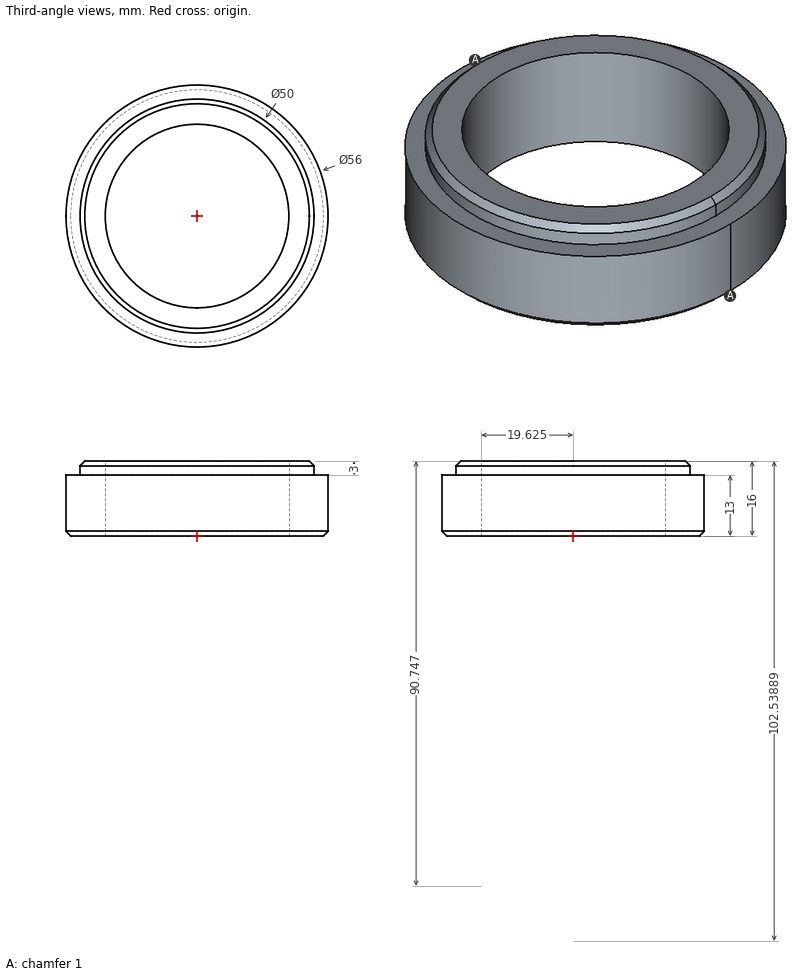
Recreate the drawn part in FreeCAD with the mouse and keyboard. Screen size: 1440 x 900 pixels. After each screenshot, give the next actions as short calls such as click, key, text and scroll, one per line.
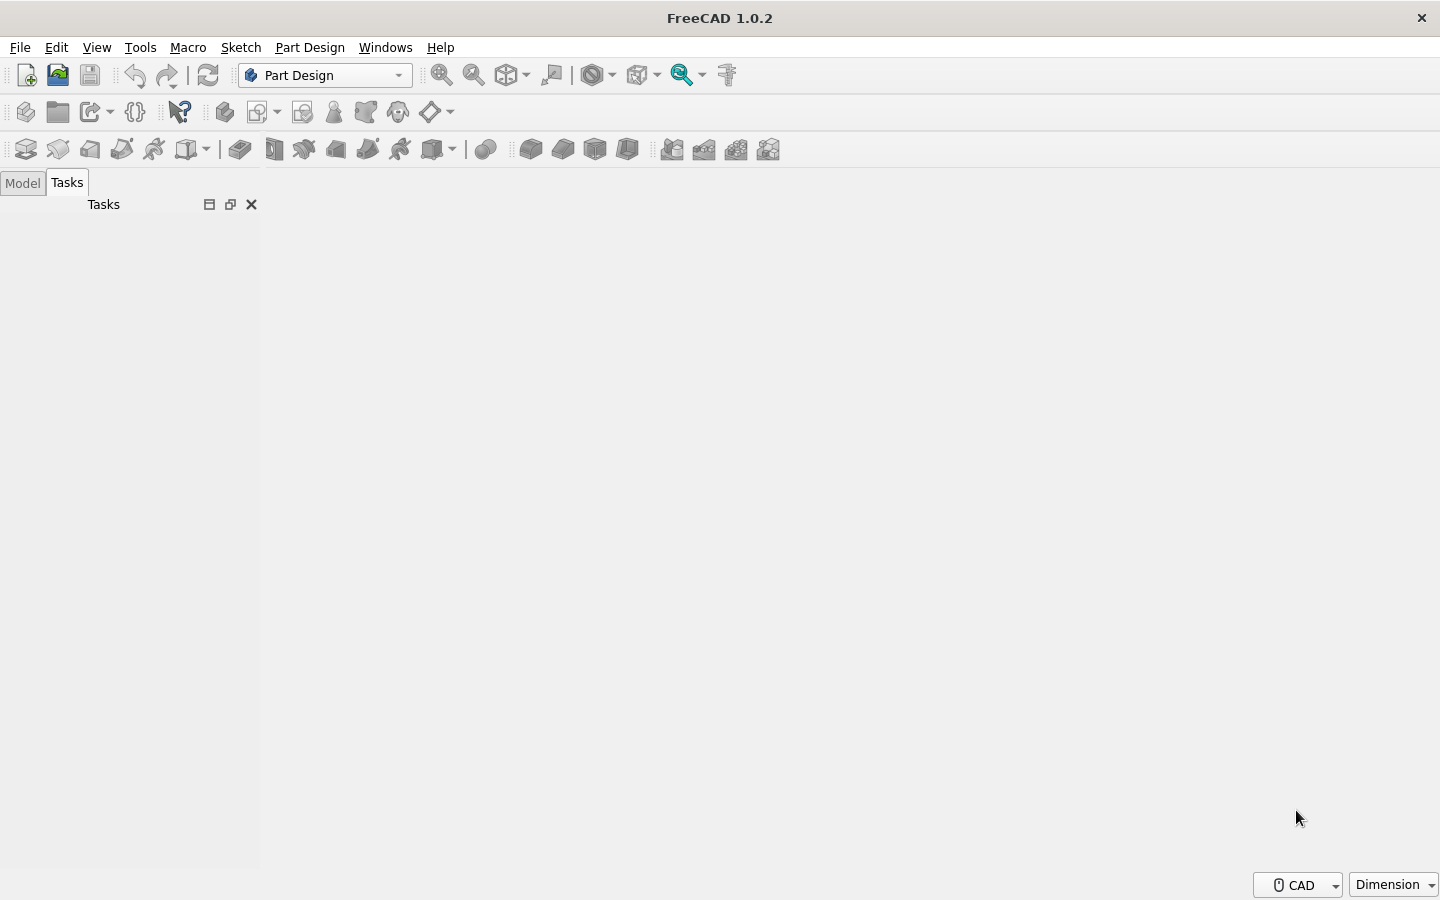
click(290, 76)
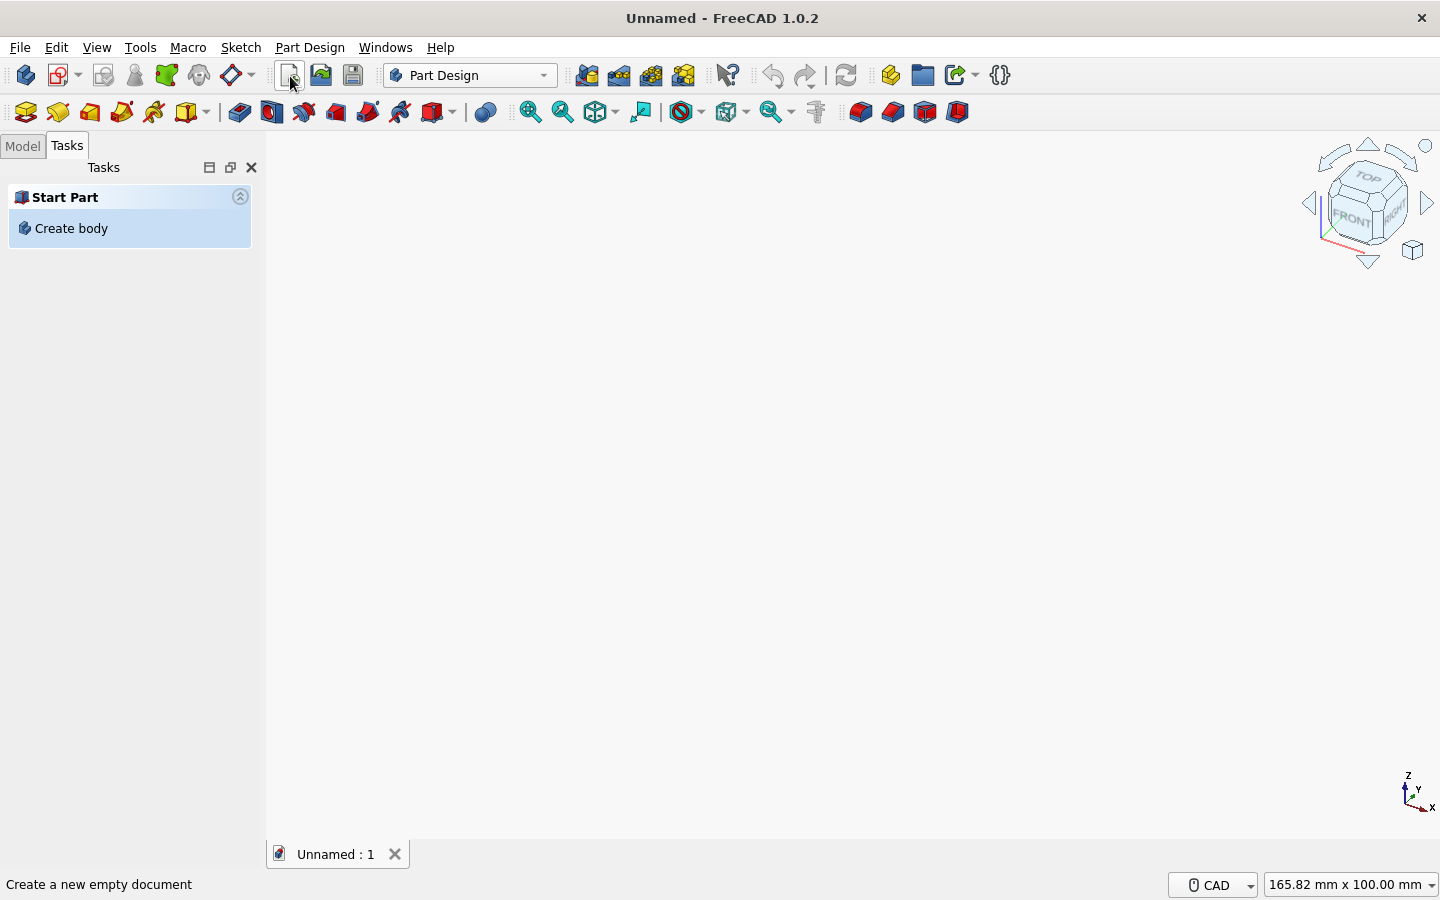
click(58, 76)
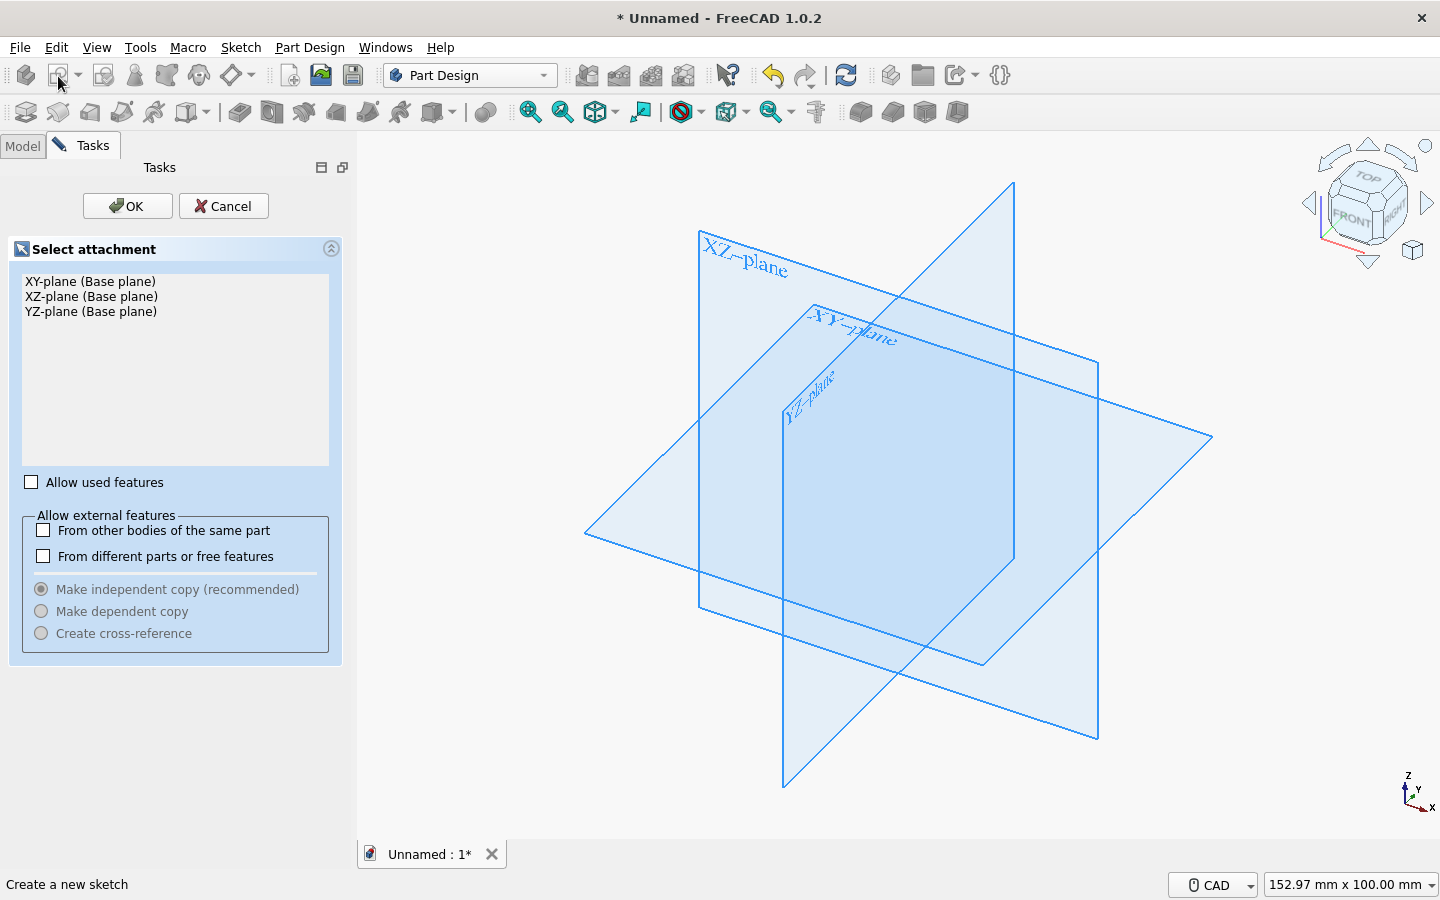
click(82, 282)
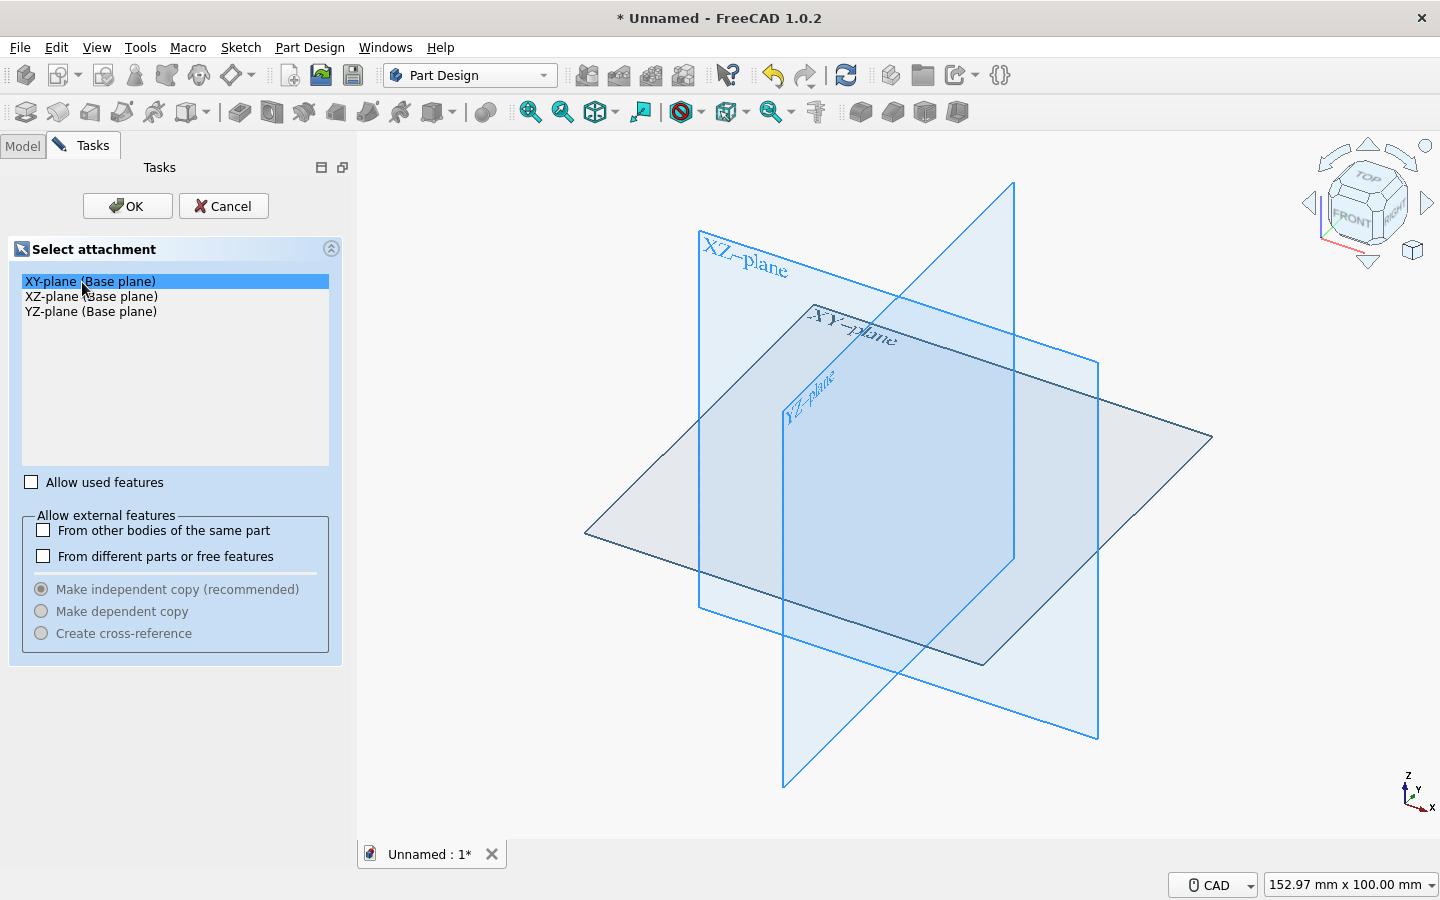
click(128, 206)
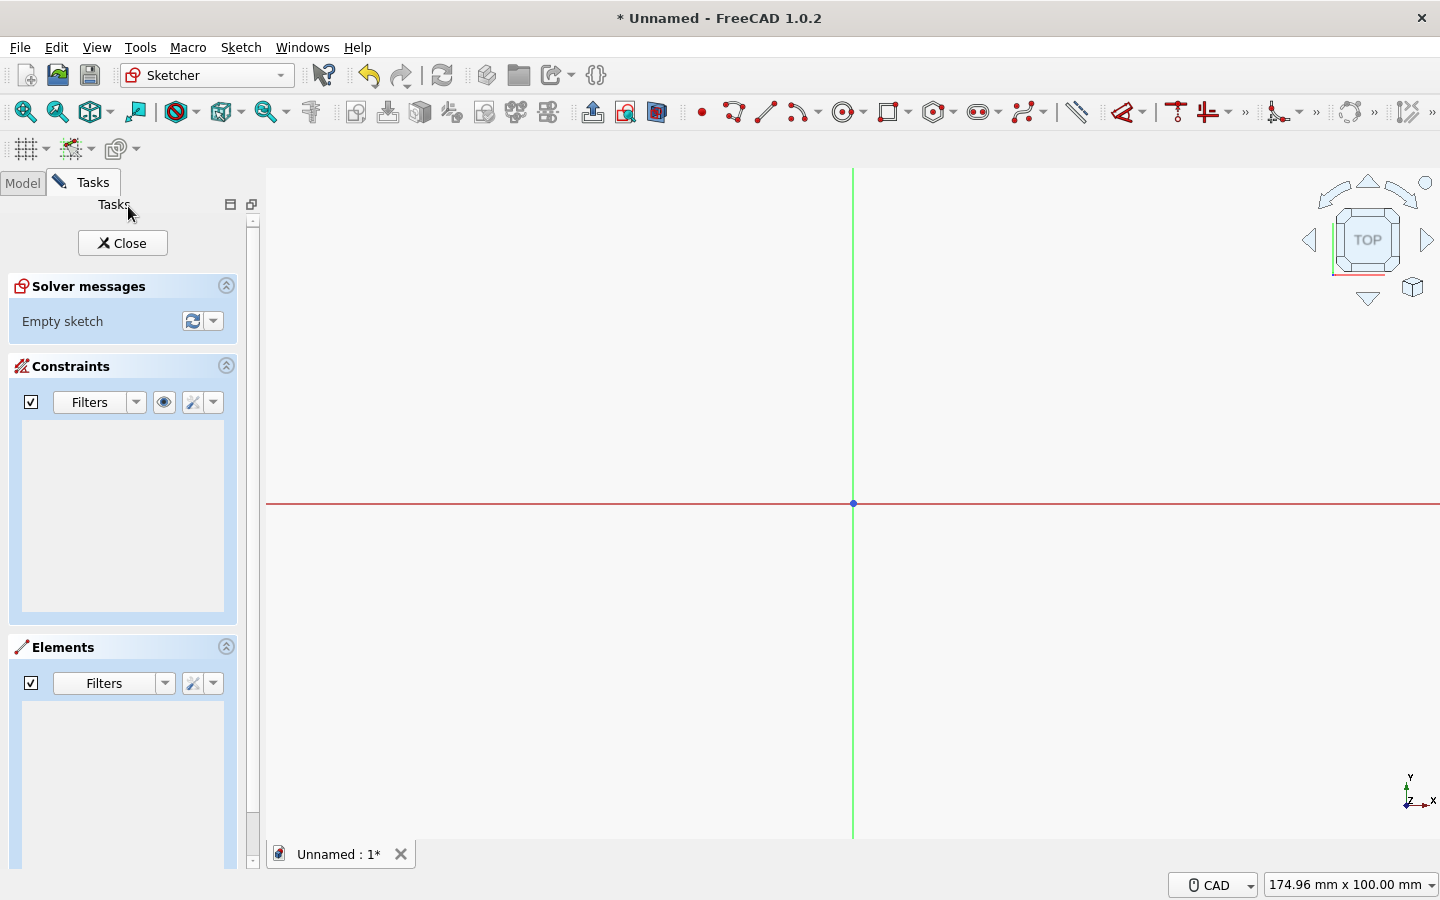
click(844, 112)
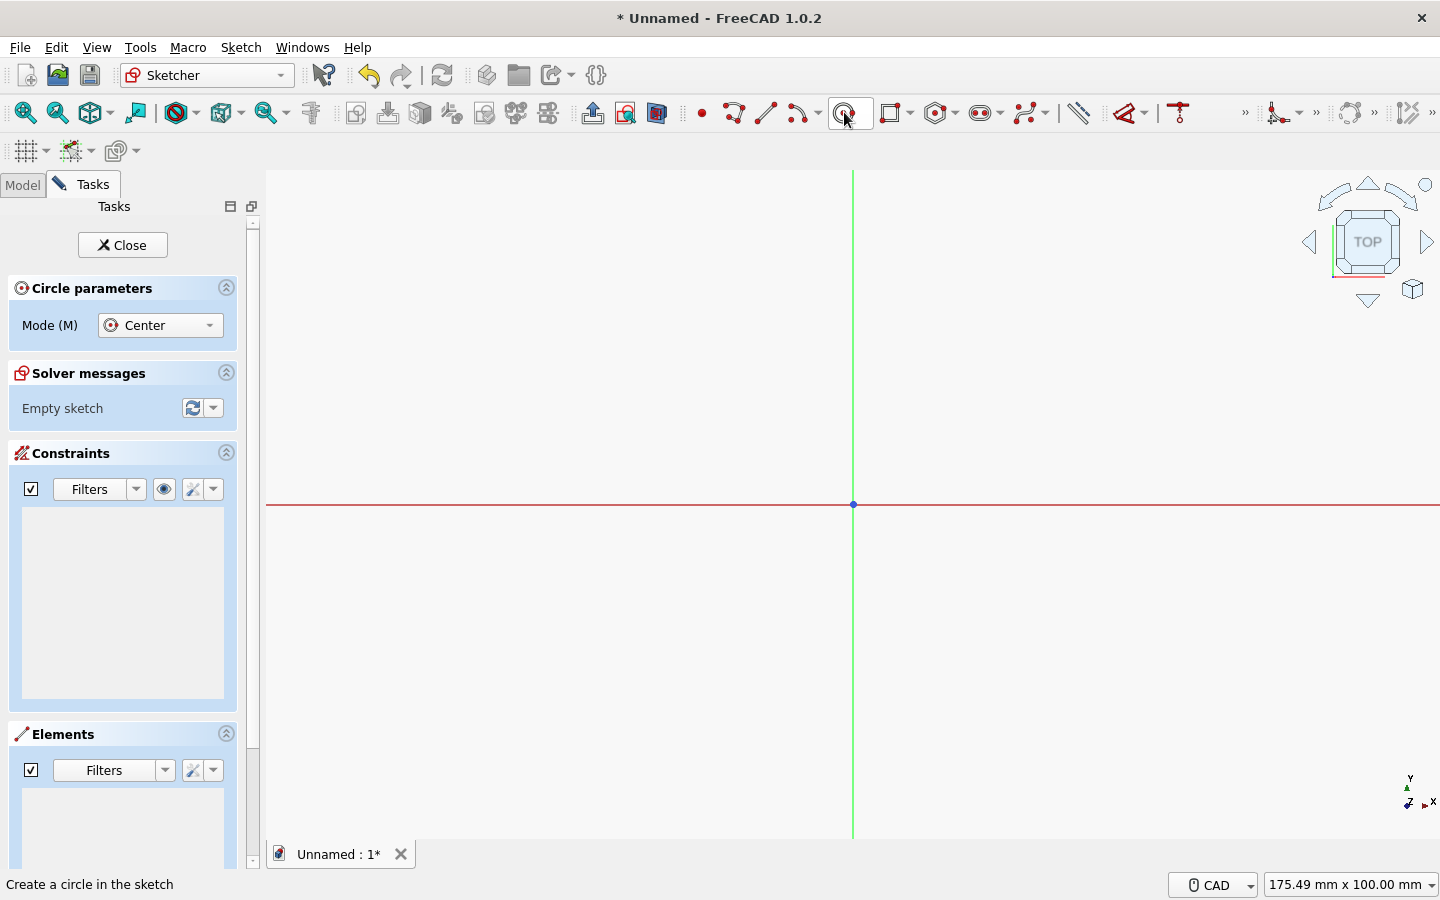
click(853, 504)
move(985, 372)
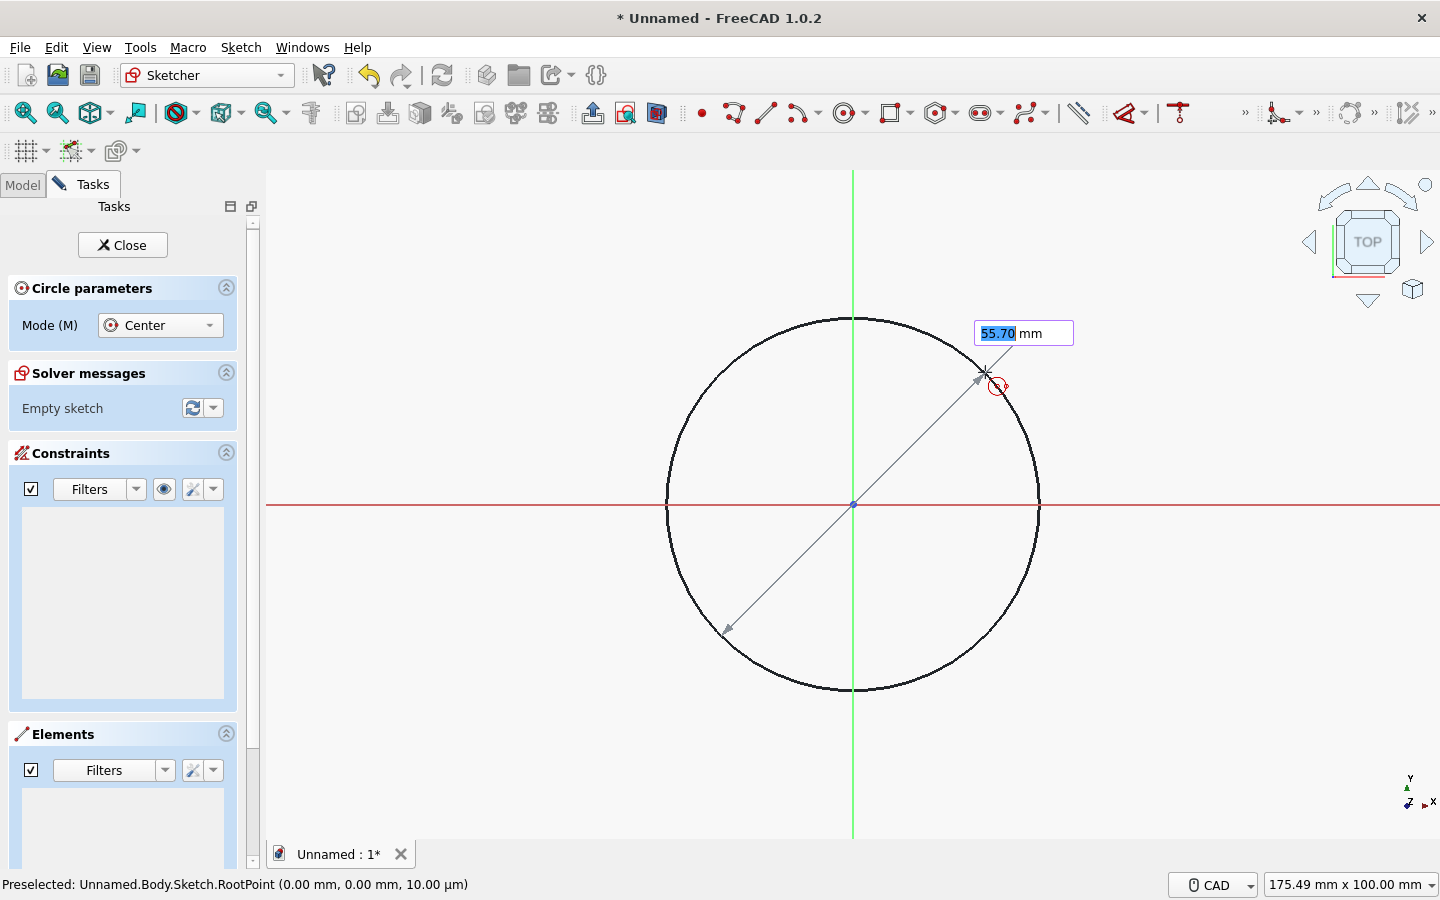
text(56)
key(Return)
key(Escape)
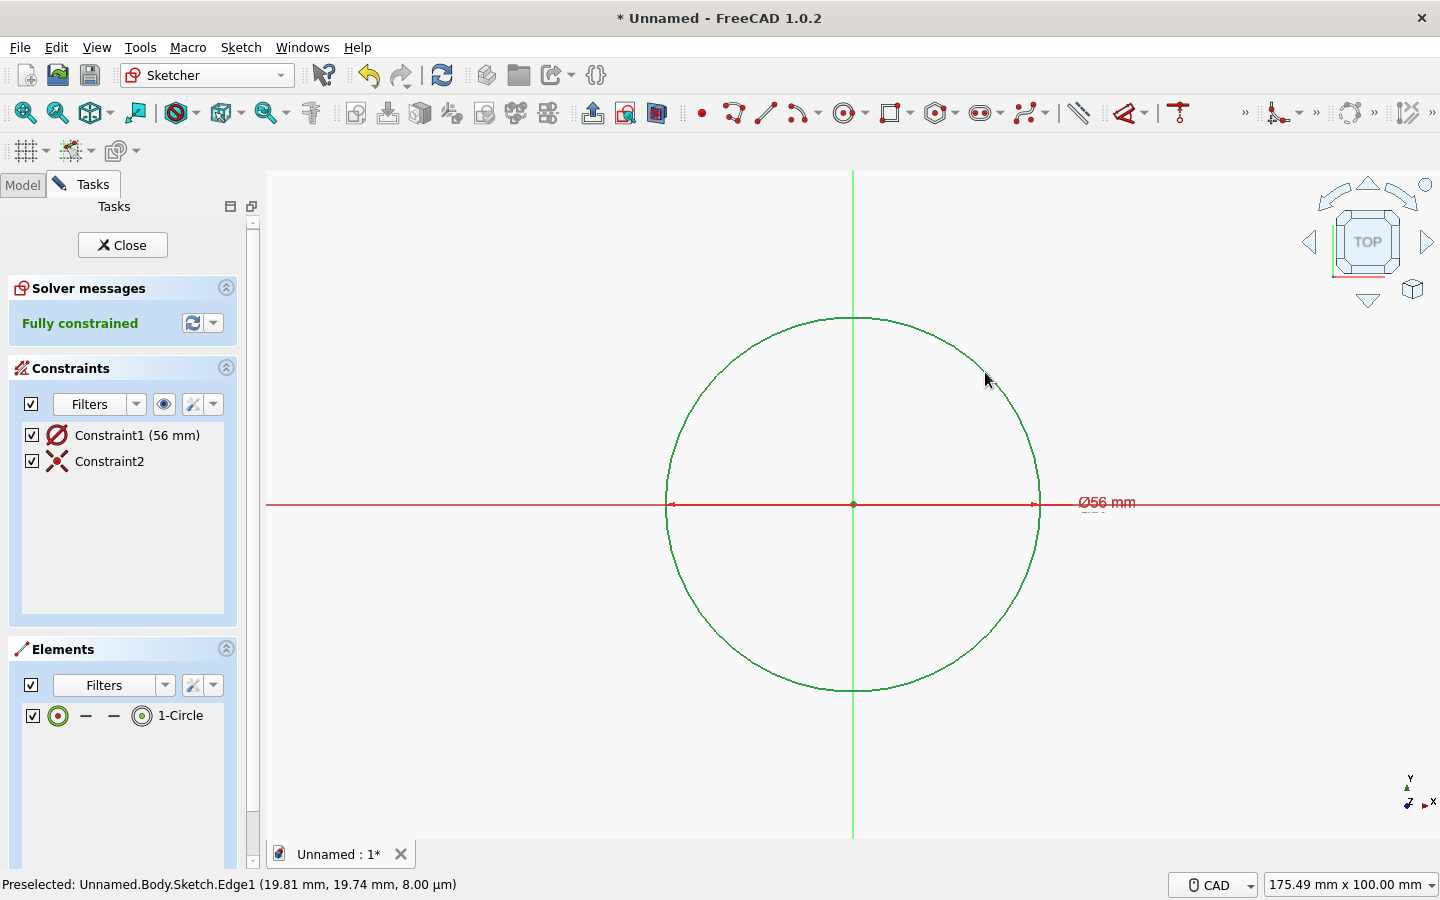
click(123, 245)